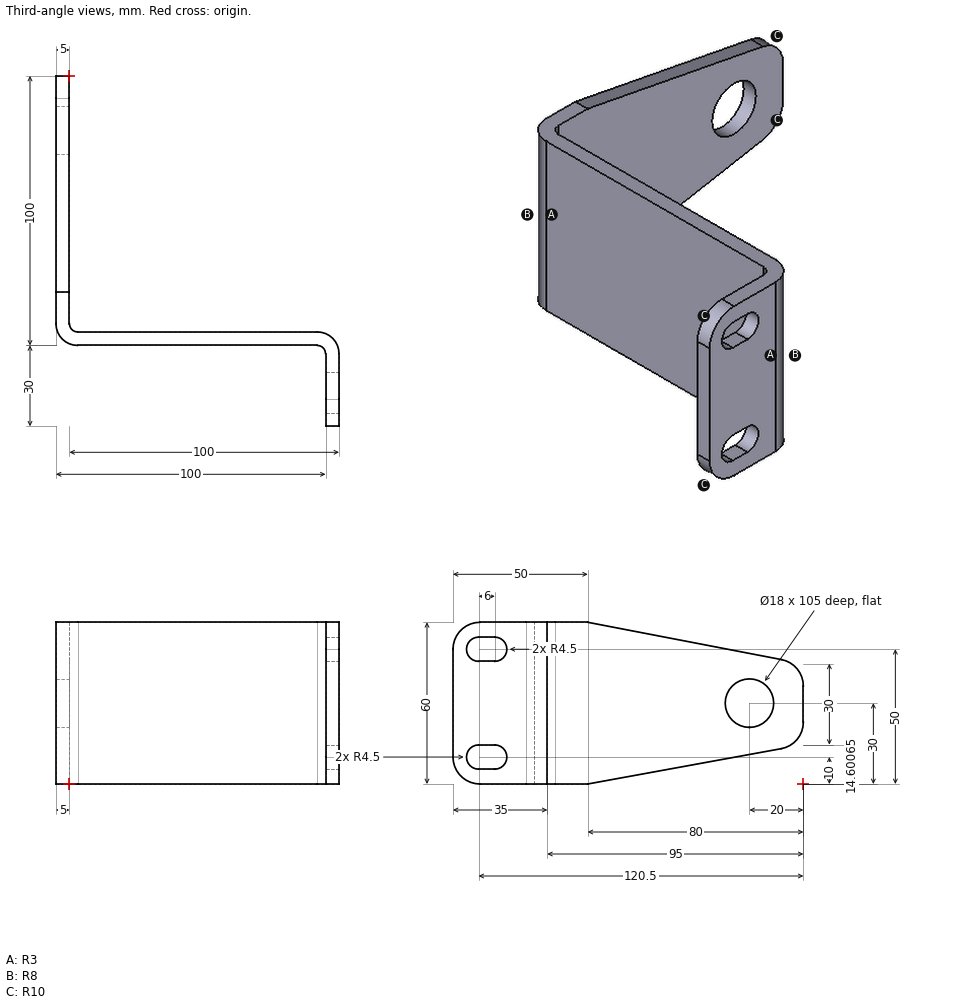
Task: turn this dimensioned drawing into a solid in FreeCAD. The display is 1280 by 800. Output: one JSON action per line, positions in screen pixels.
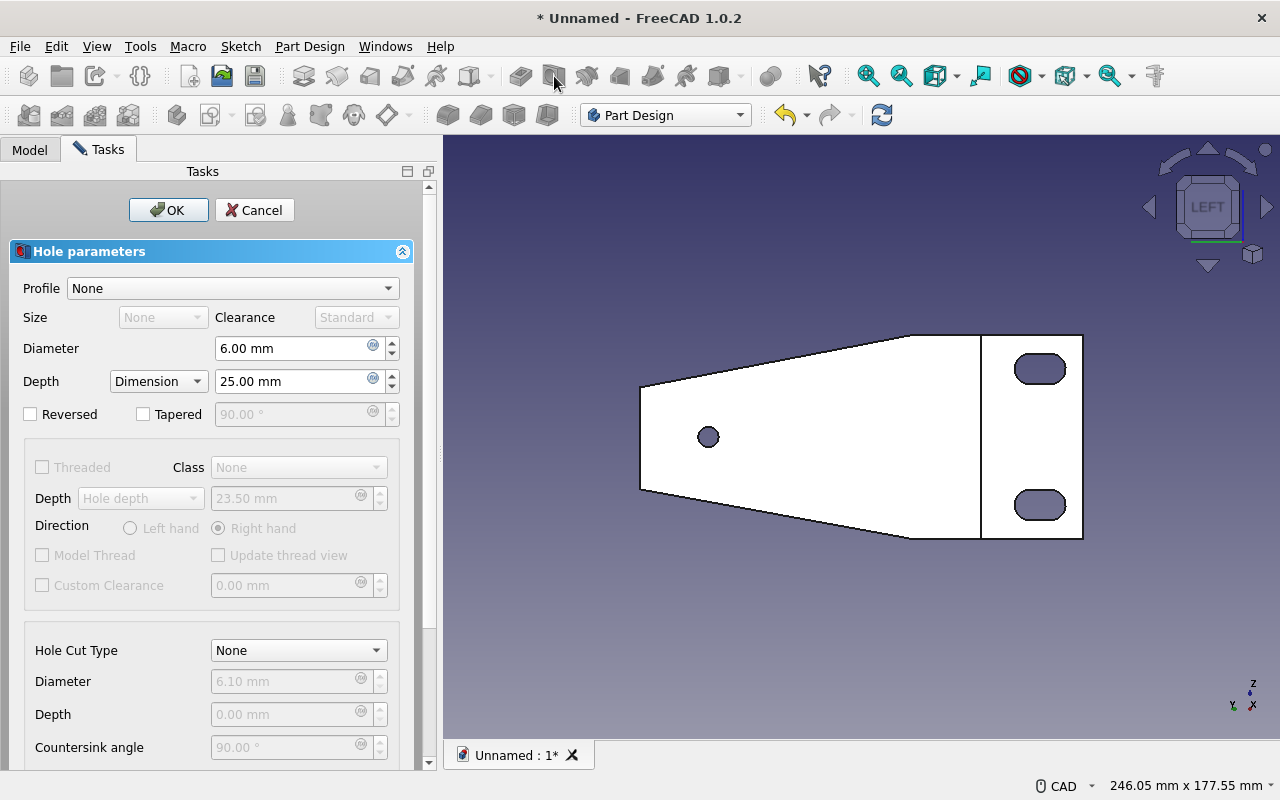
{"action": "triple_click", "coordinate": [300, 348]}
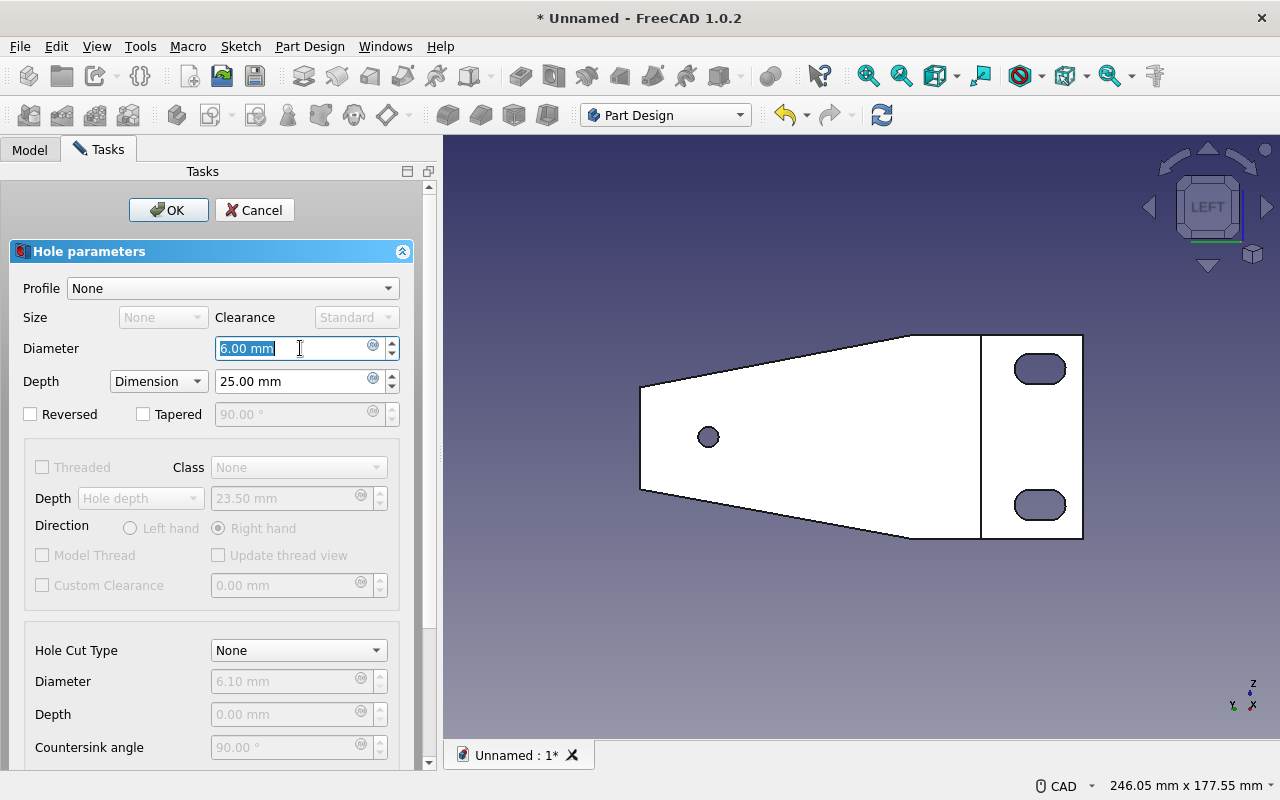
{"action": "type", "text": "18"}
{"action": "key", "text": "Tab"}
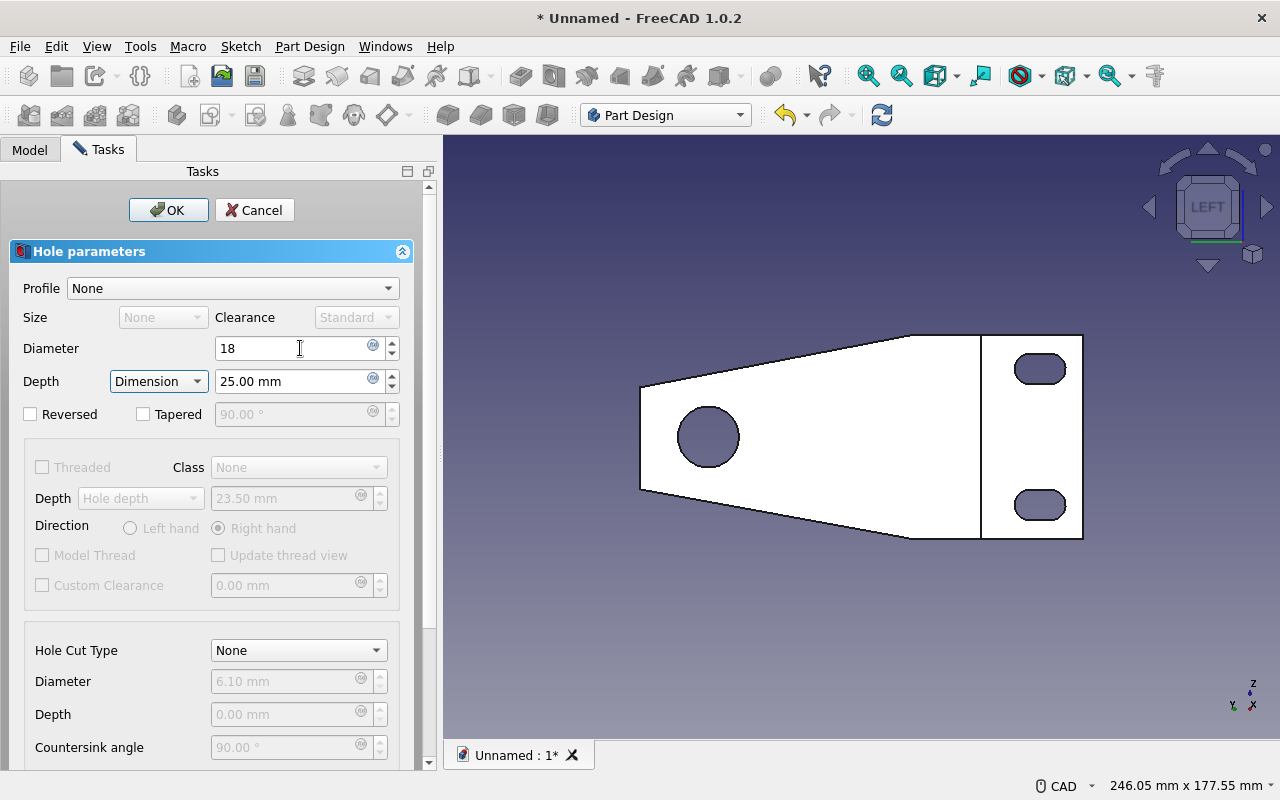
{"action": "triple_click", "coordinate": [300, 382]}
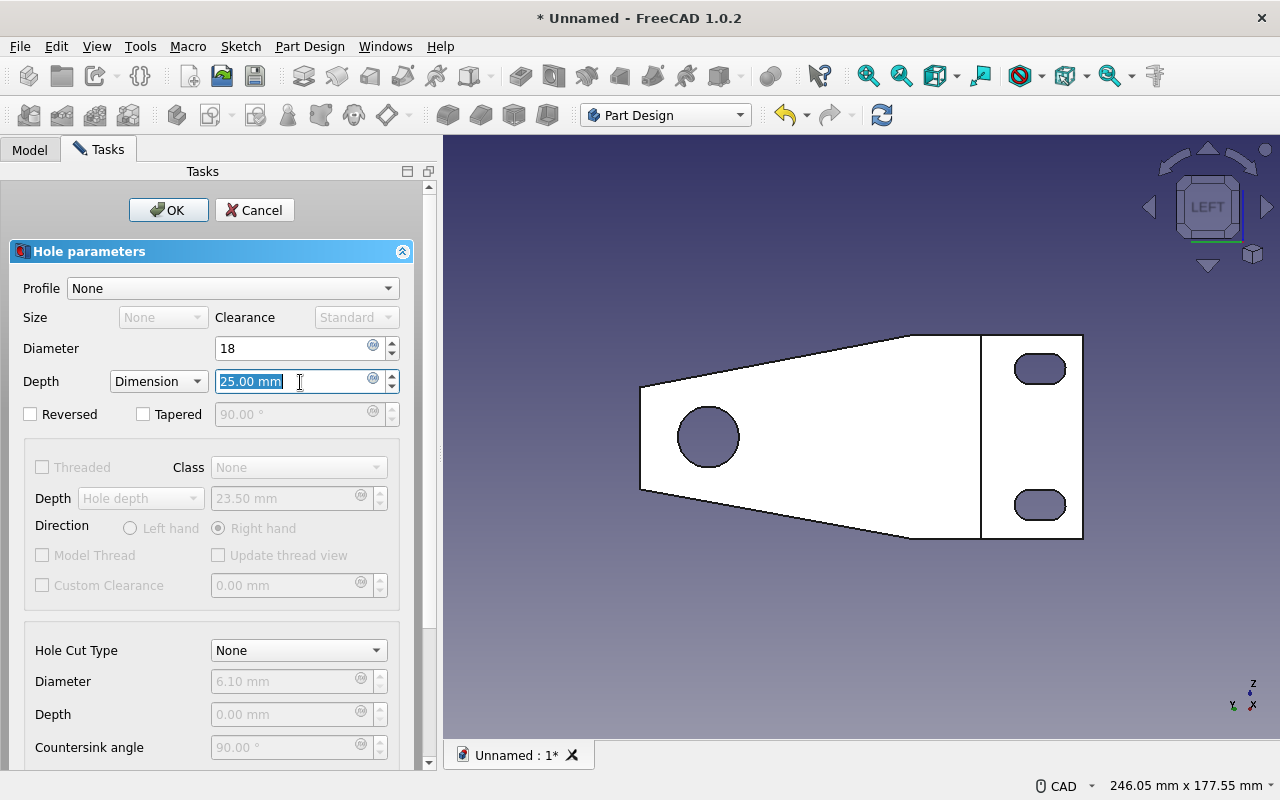
{"action": "type", "text": "105"}
{"action": "key", "text": "Tab"}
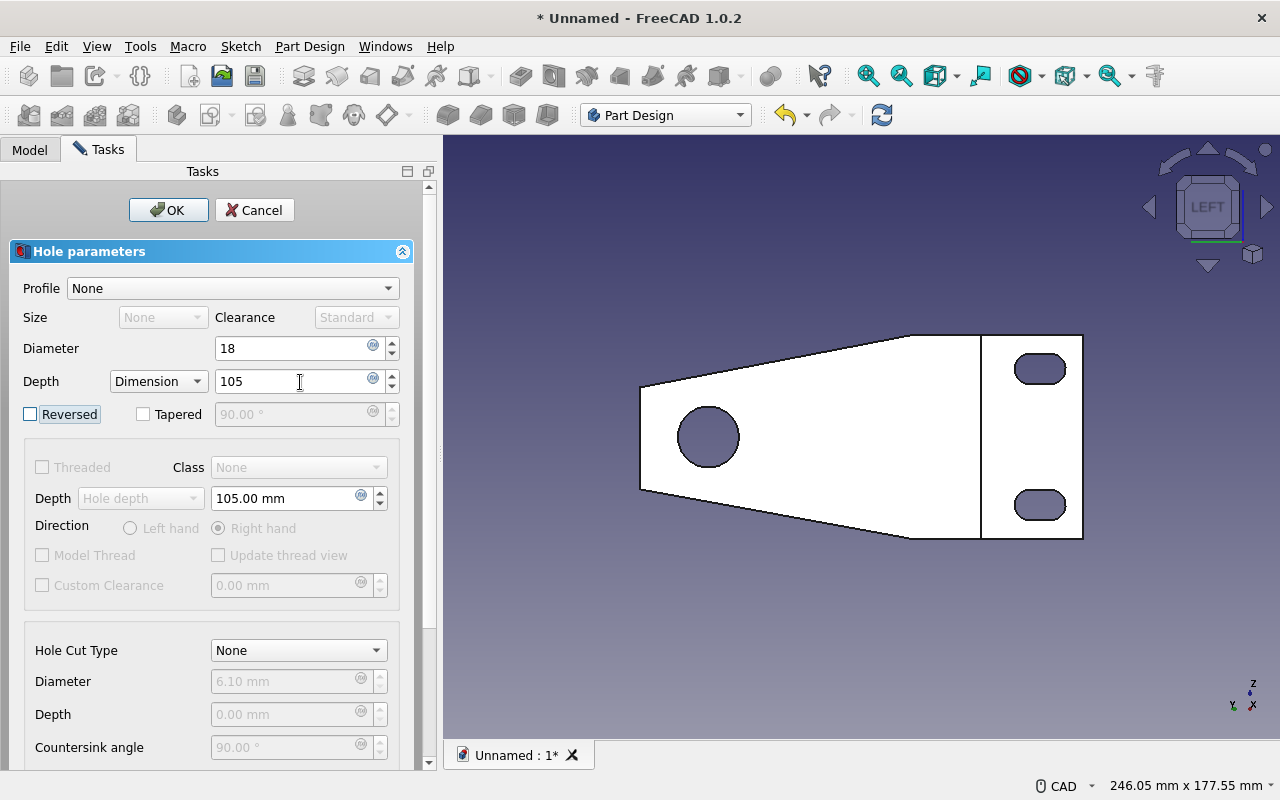
{"action": "scroll", "coordinate": [429, 476], "scroll_direction": "down", "scroll_amount": 3}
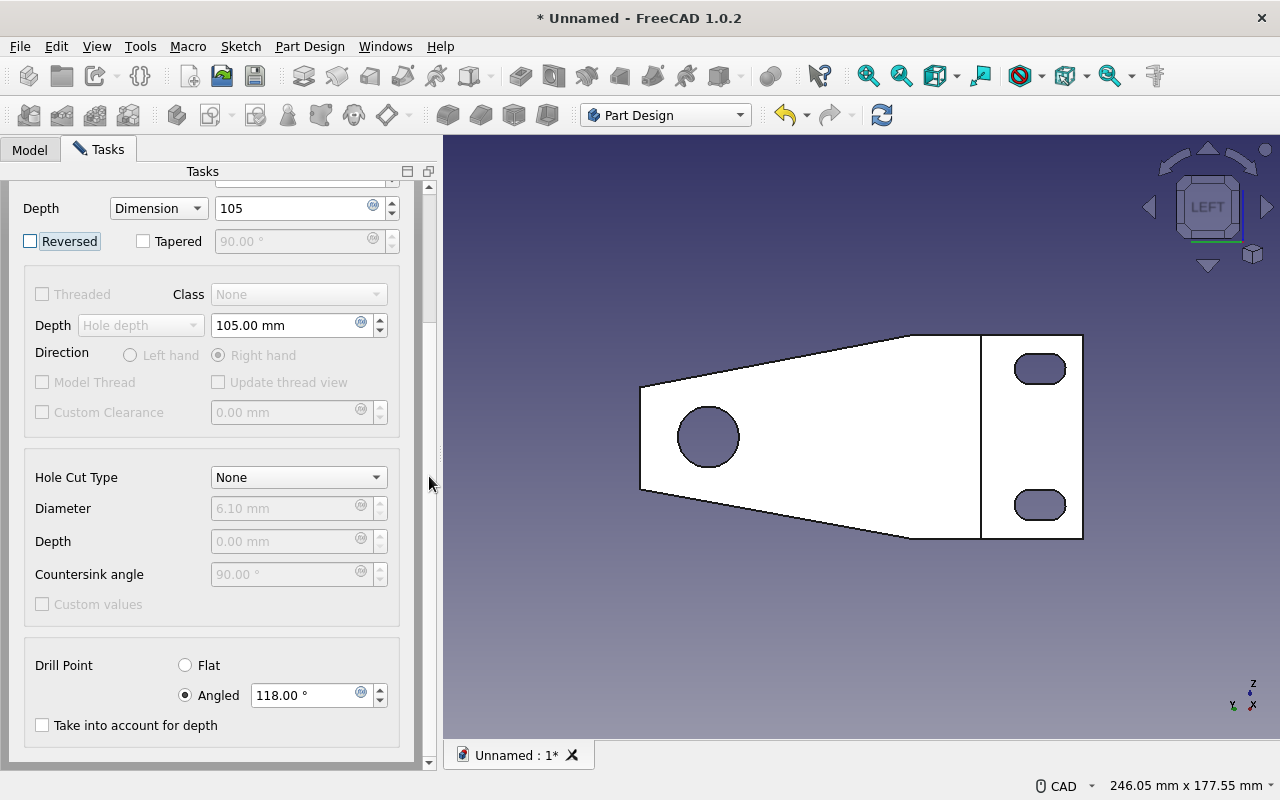
{"action": "left_click", "coordinate": [186, 663]}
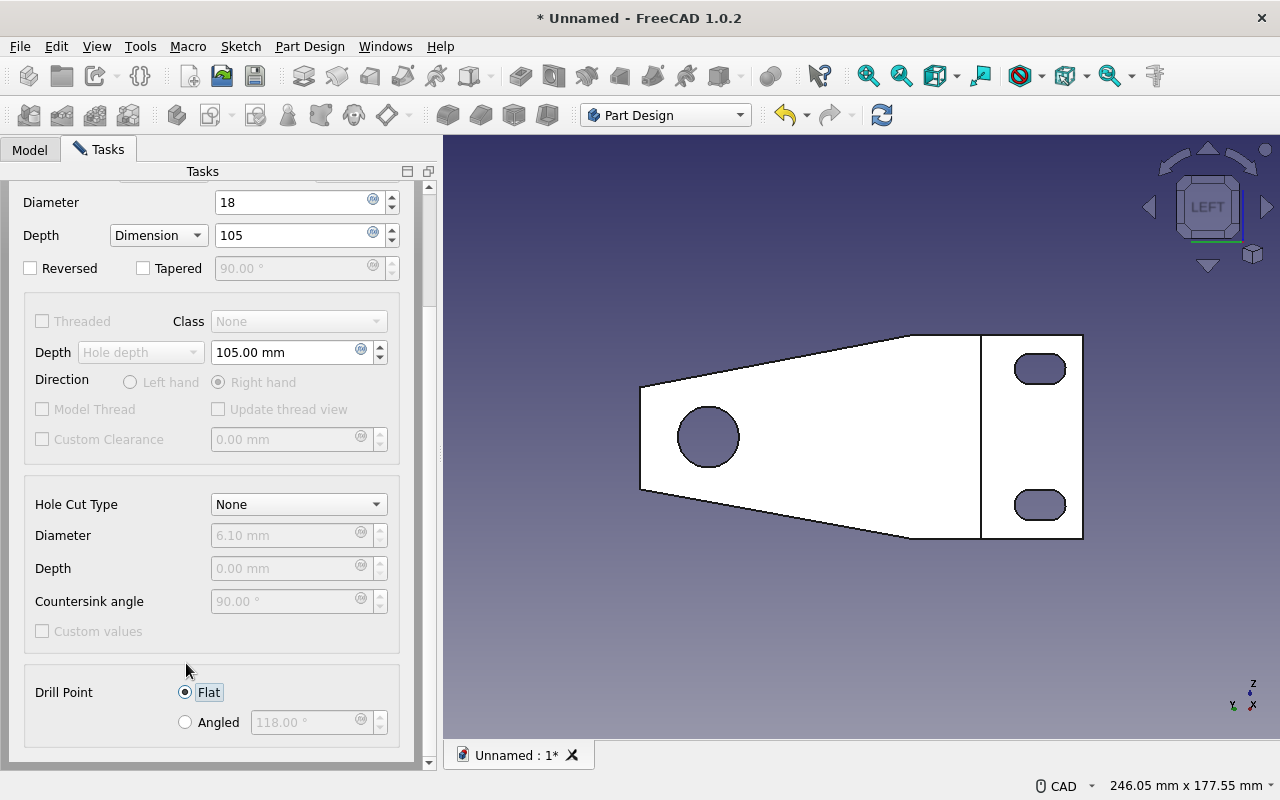
{"action": "scroll", "coordinate": [429, 476], "scroll_direction": "up", "scroll_amount": 4}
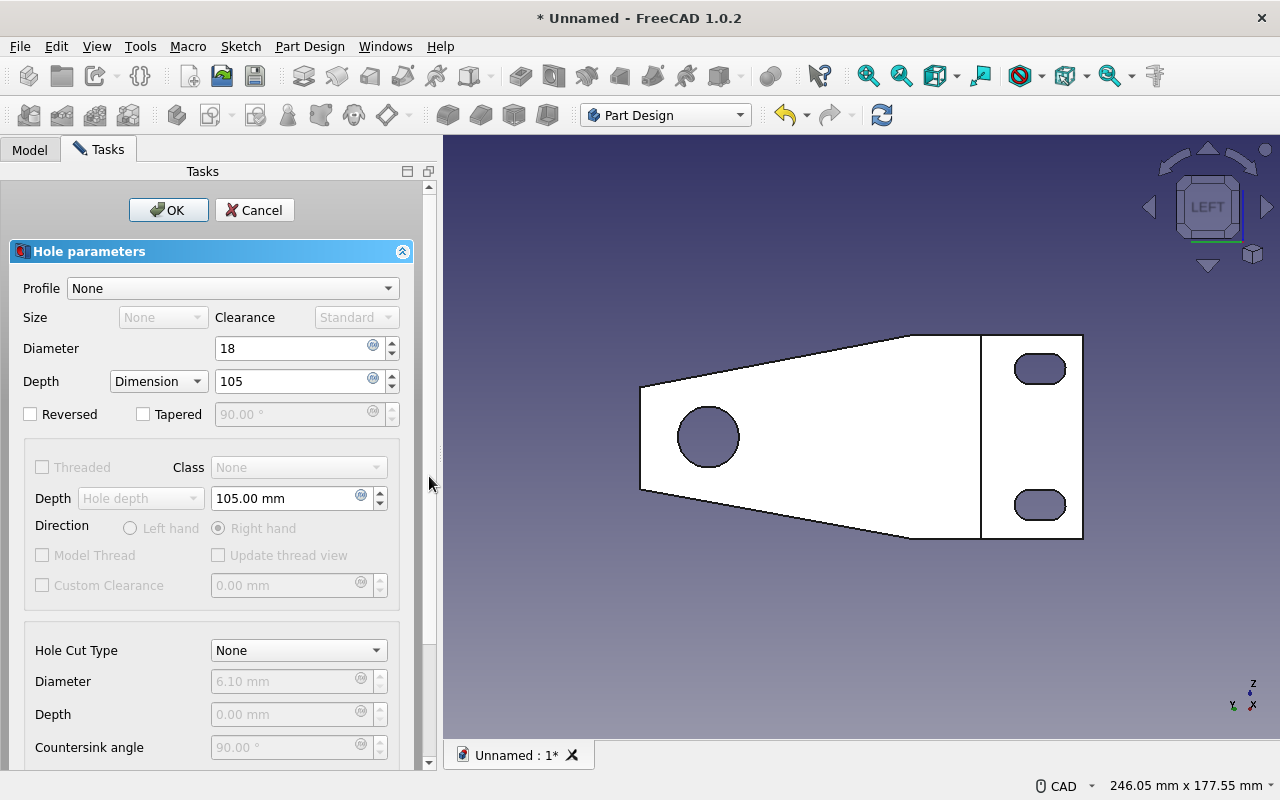
{"action": "left_click", "coordinate": [169, 210]}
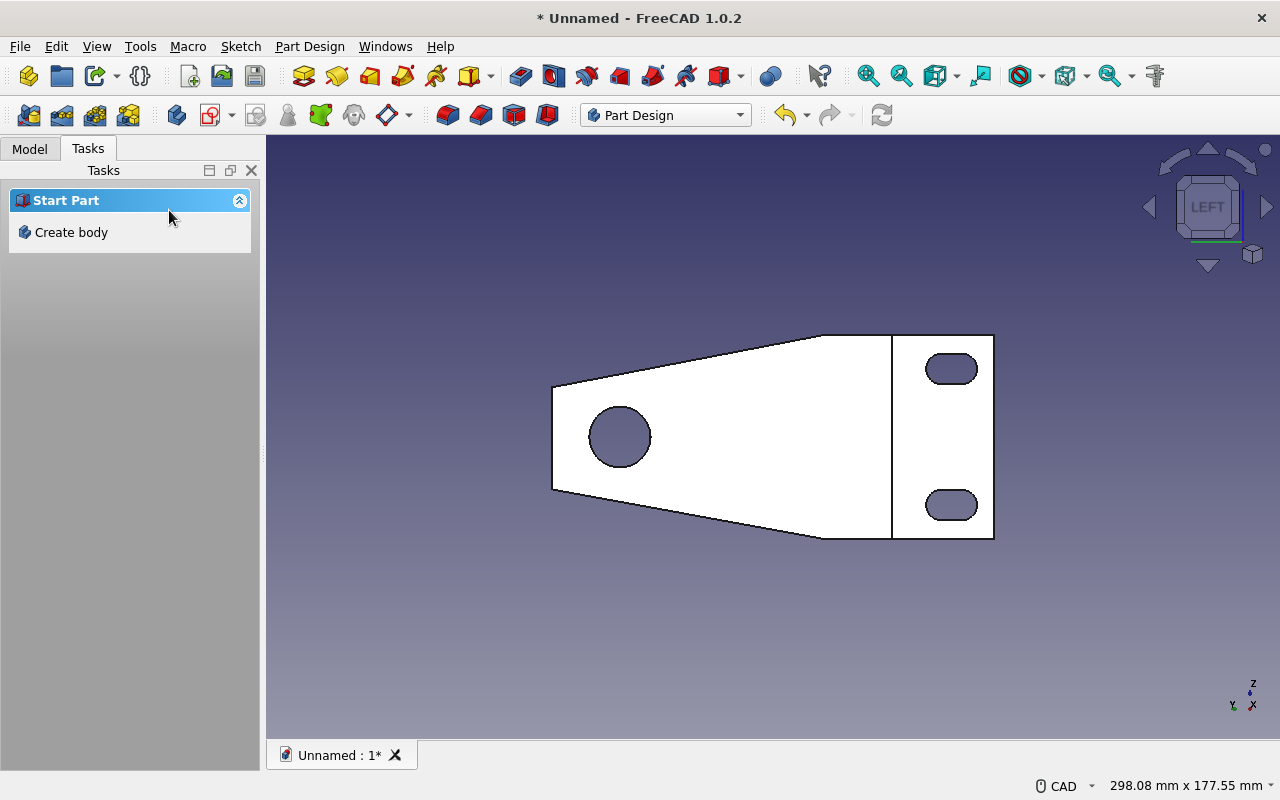
{"action": "left_click", "coordinate": [869, 76]}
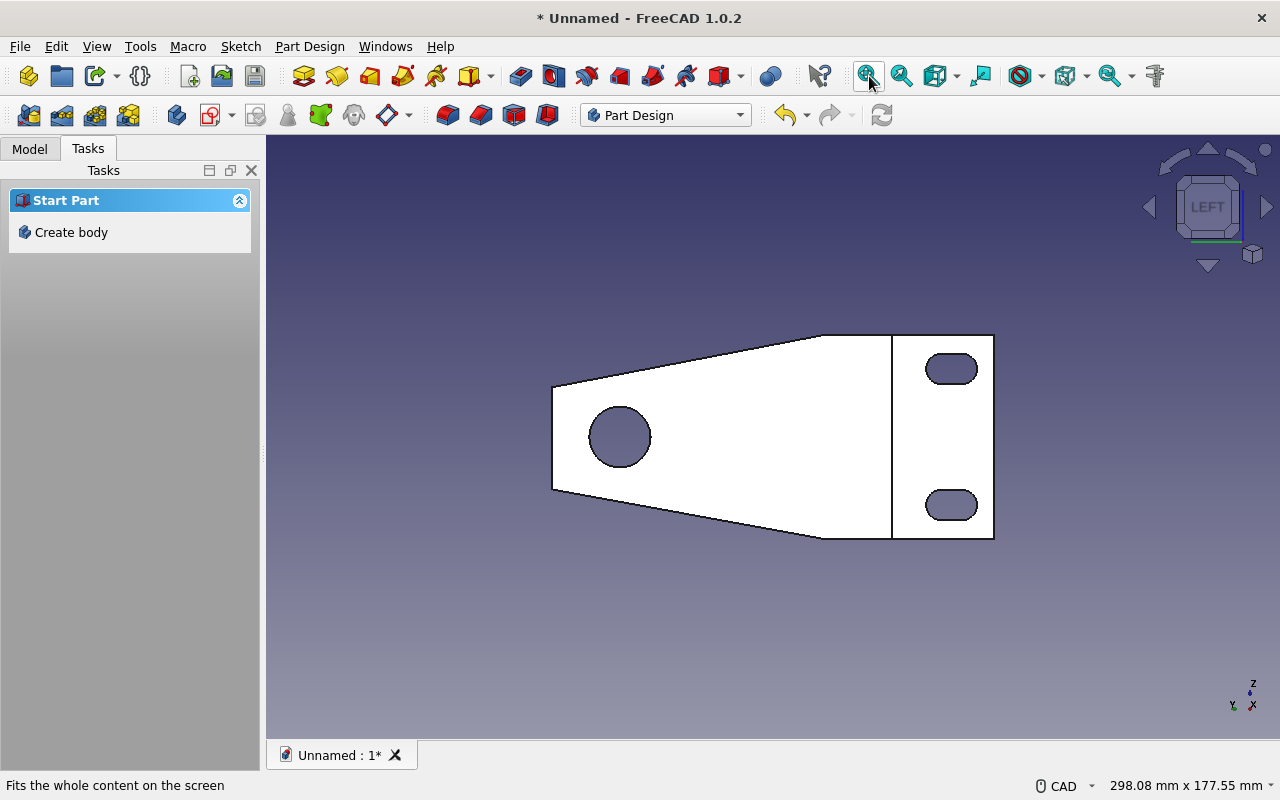
{"action": "key", "text": "0"}